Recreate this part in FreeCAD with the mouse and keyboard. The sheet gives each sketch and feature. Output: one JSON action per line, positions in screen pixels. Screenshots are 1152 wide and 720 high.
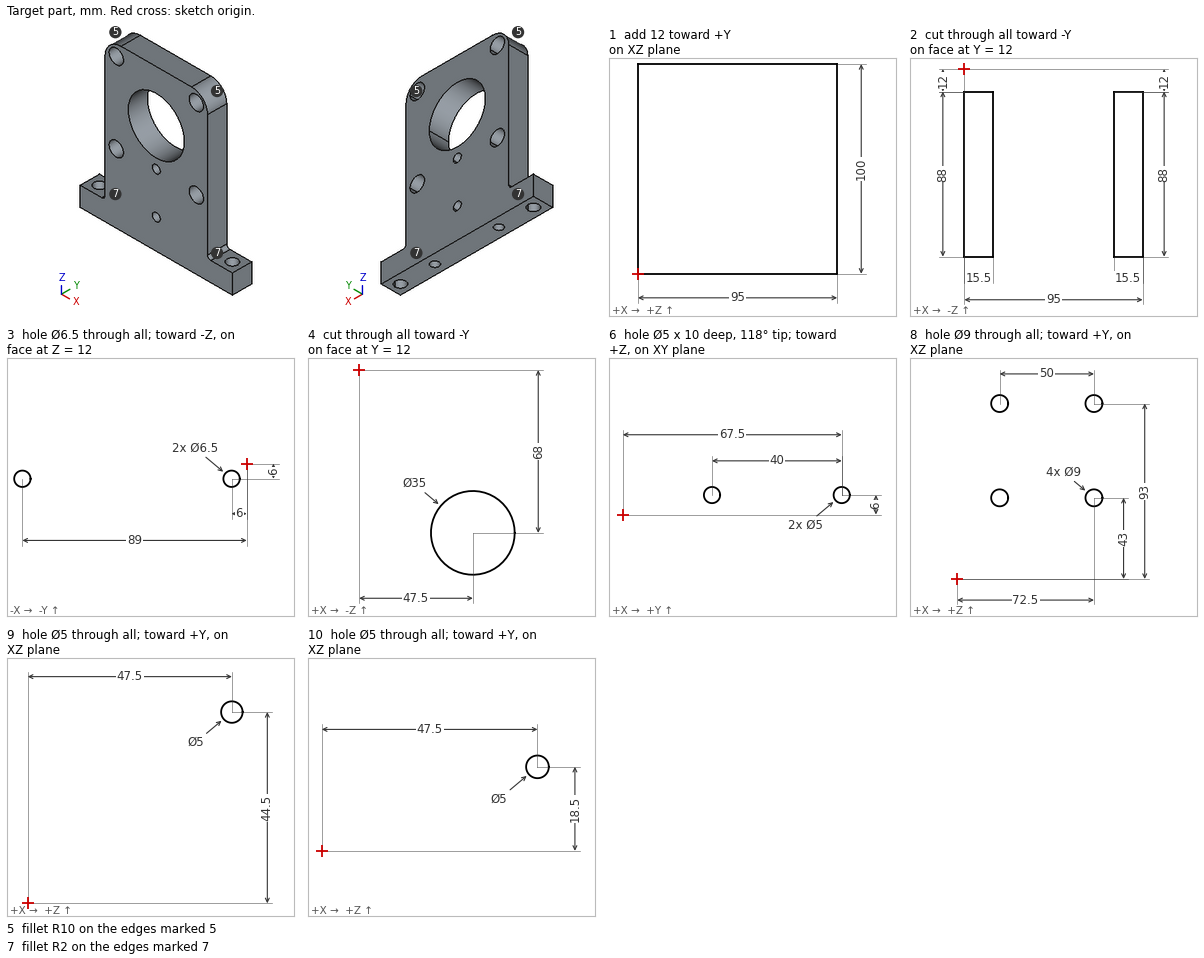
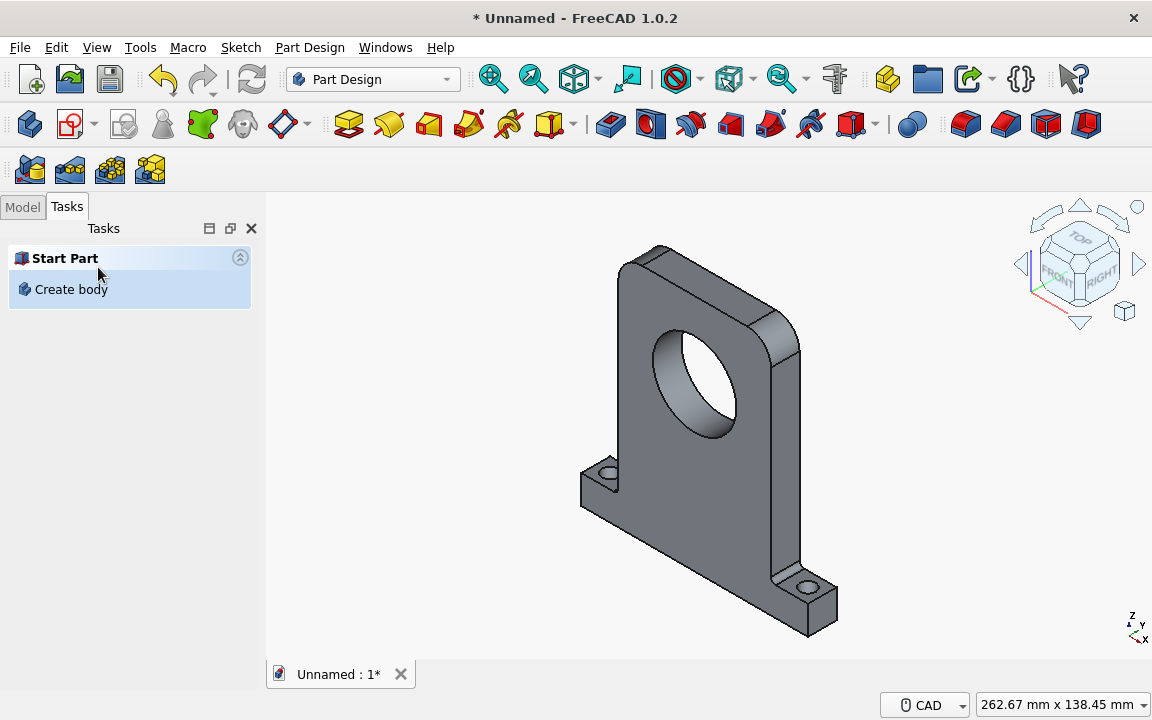
{"action": "left_click", "coordinate": [70, 124]}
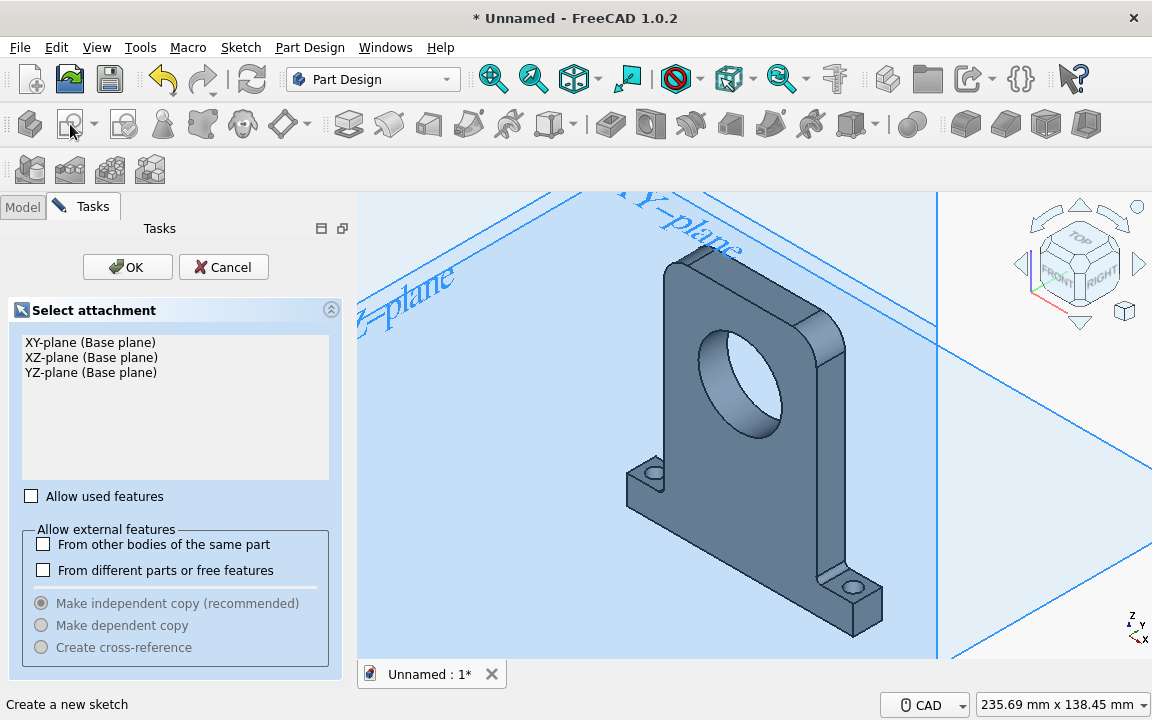
{"action": "left_click", "coordinate": [82, 358]}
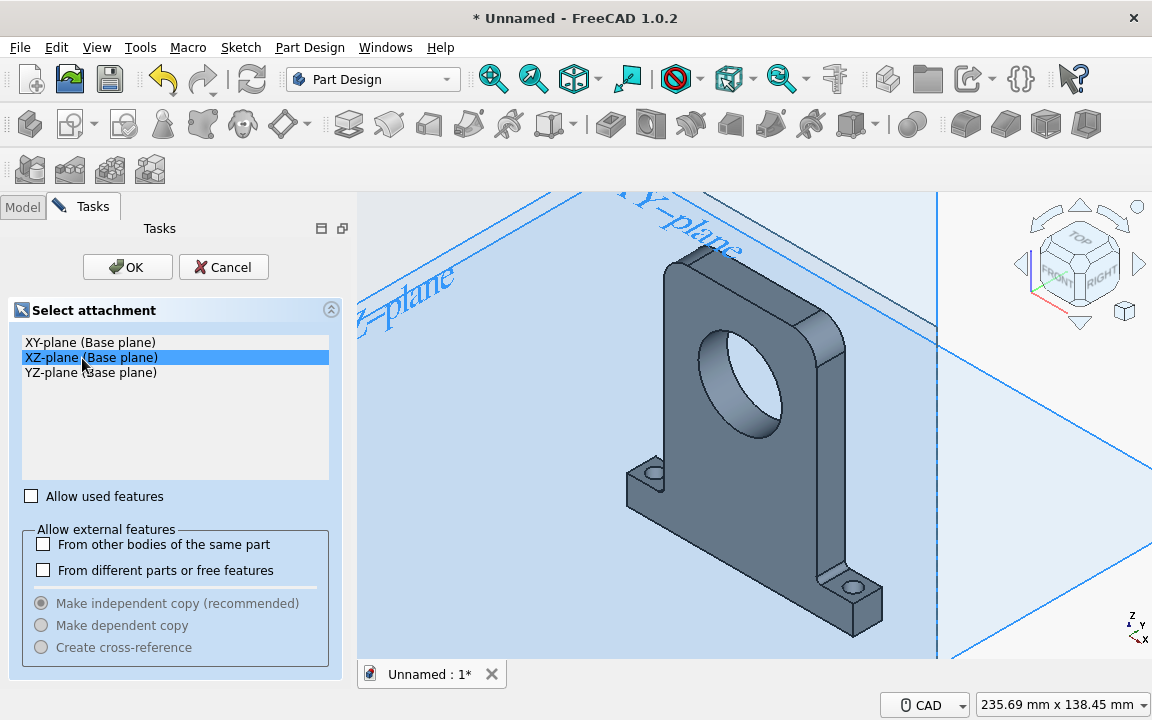
{"action": "left_click", "coordinate": [128, 267]}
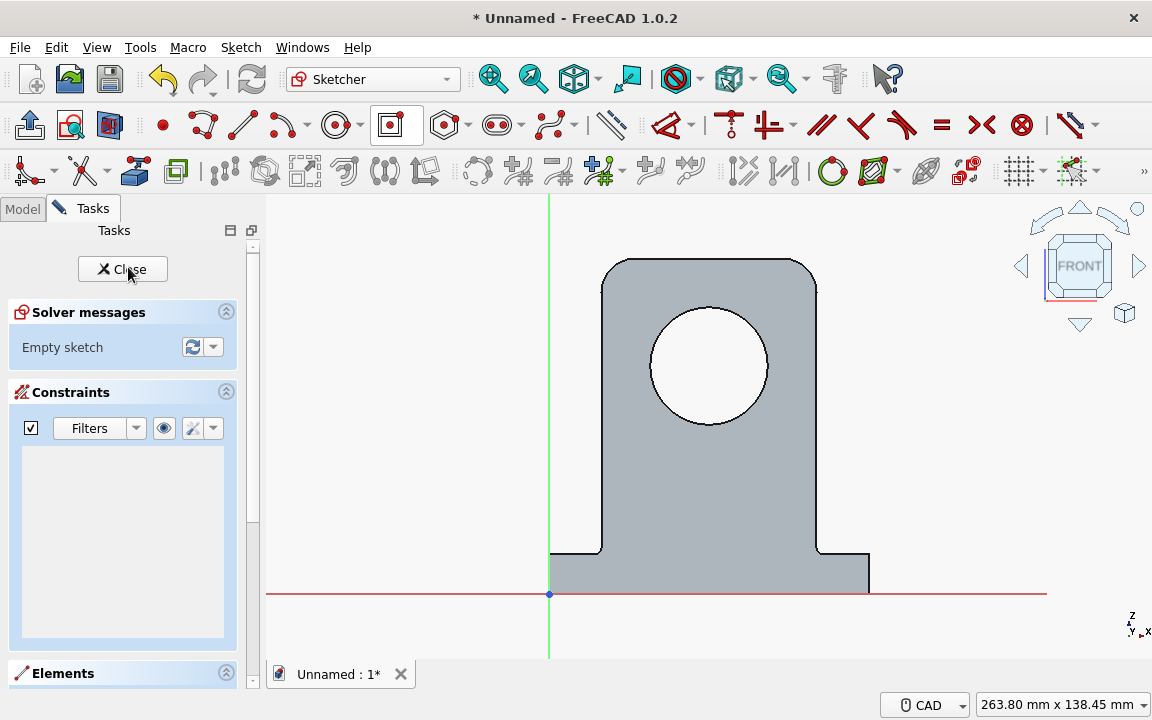
{"action": "left_click", "coordinate": [336, 126]}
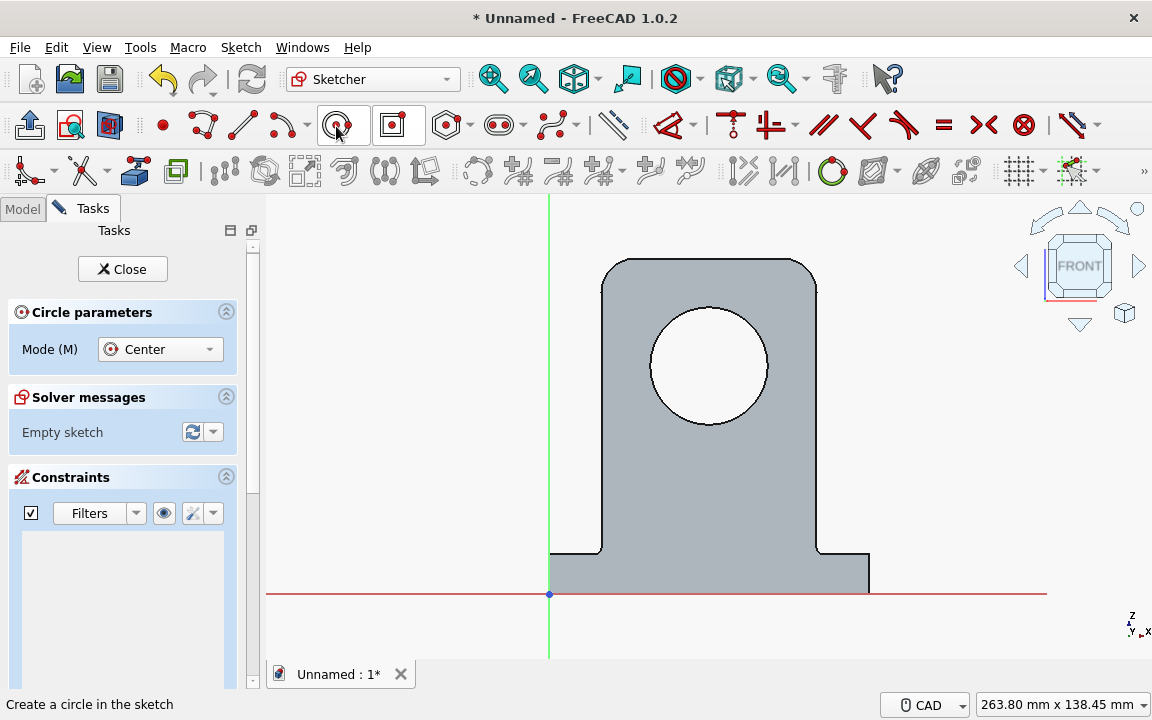
{"action": "scroll", "coordinate": [793, 450], "scroll_direction": "up", "scroll_amount": 3}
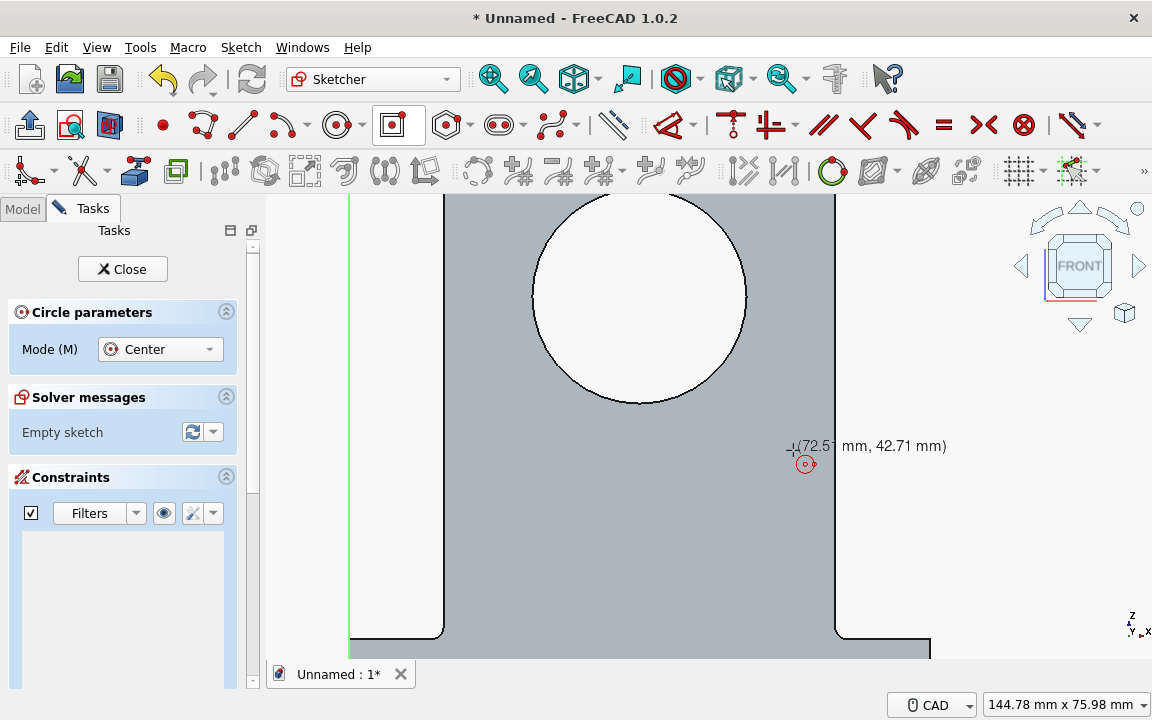
{"action": "left_click", "coordinate": [792, 450]}
{"action": "left_click", "coordinate": [812, 430]}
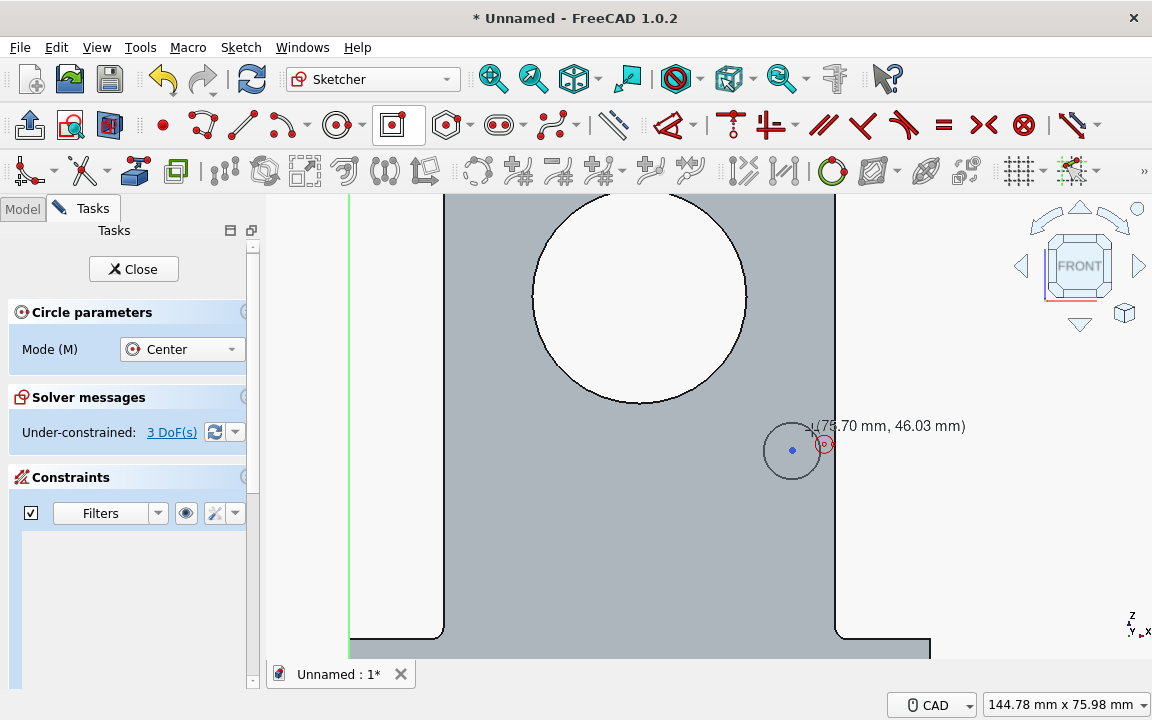
{"action": "scroll", "coordinate": [686, 436], "scroll_direction": "down", "scroll_amount": 4}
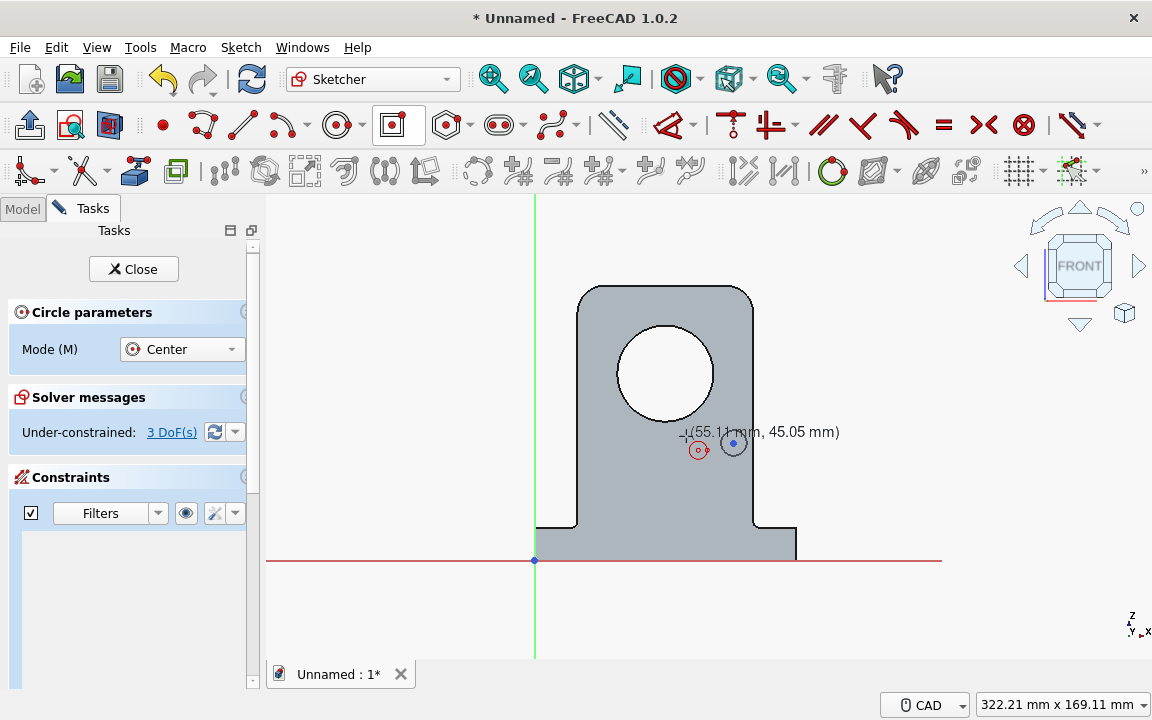
{"action": "scroll", "coordinate": [734, 305], "scroll_direction": "up", "scroll_amount": 4}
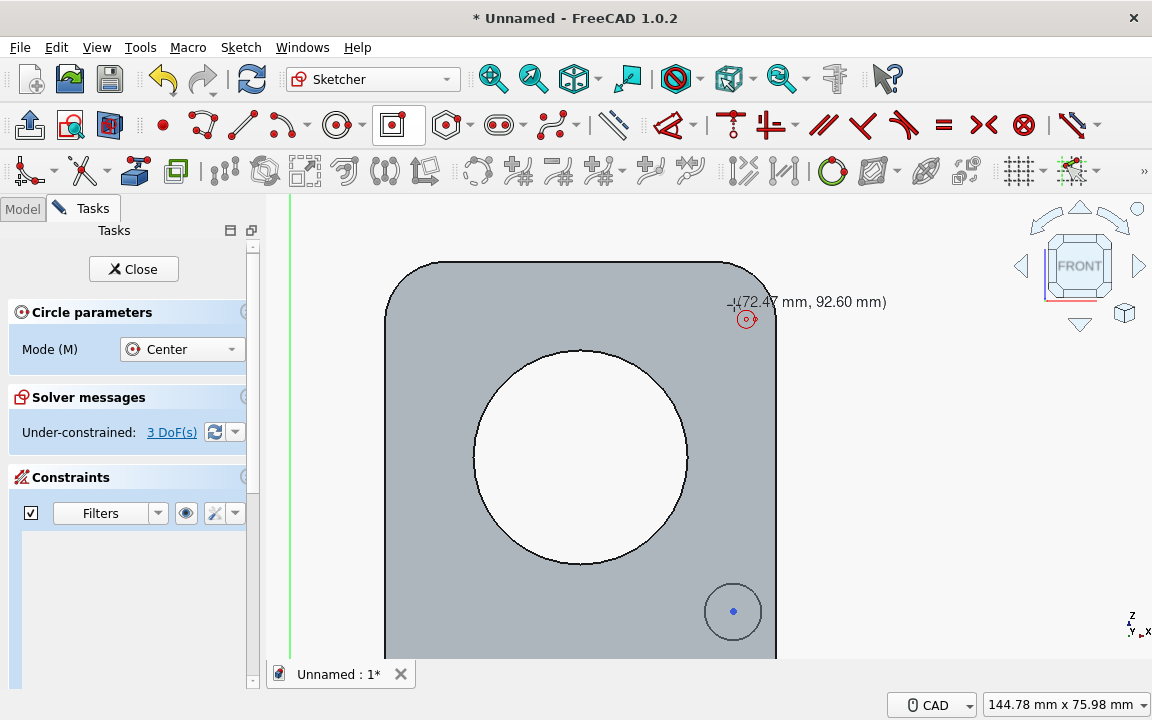
{"action": "left_click", "coordinate": [734, 304]}
{"action": "left_click", "coordinate": [753, 285]}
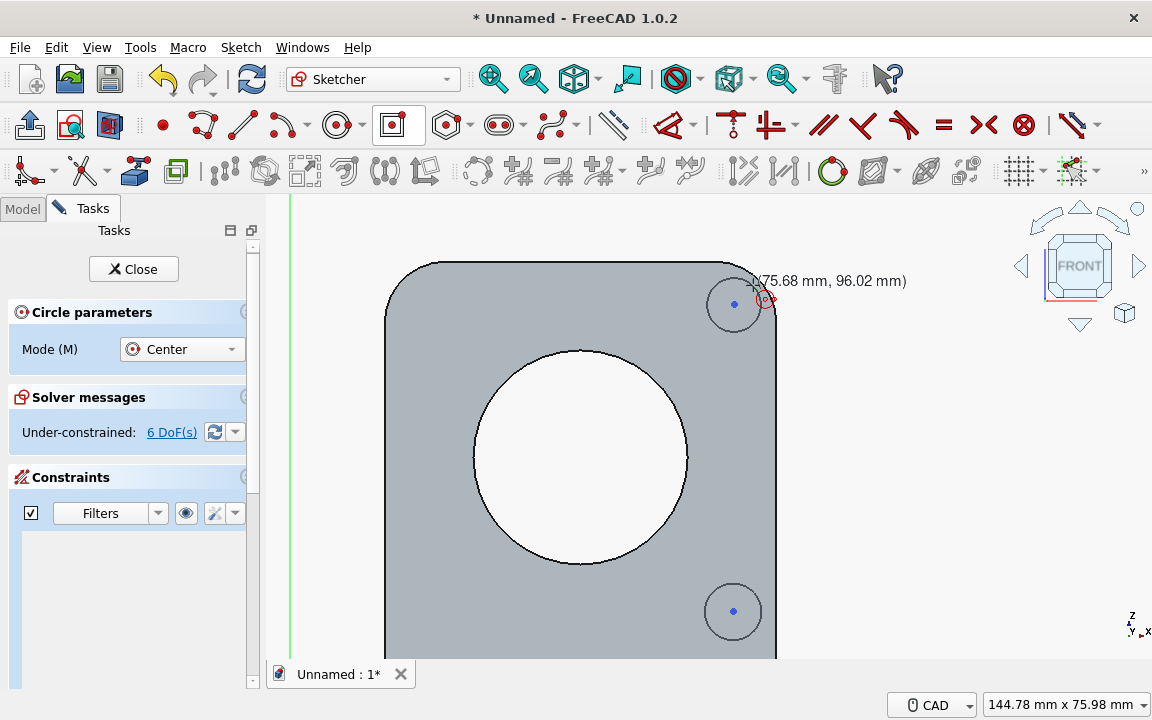
{"action": "left_click", "coordinate": [428, 304]}
{"action": "left_click", "coordinate": [447, 285]}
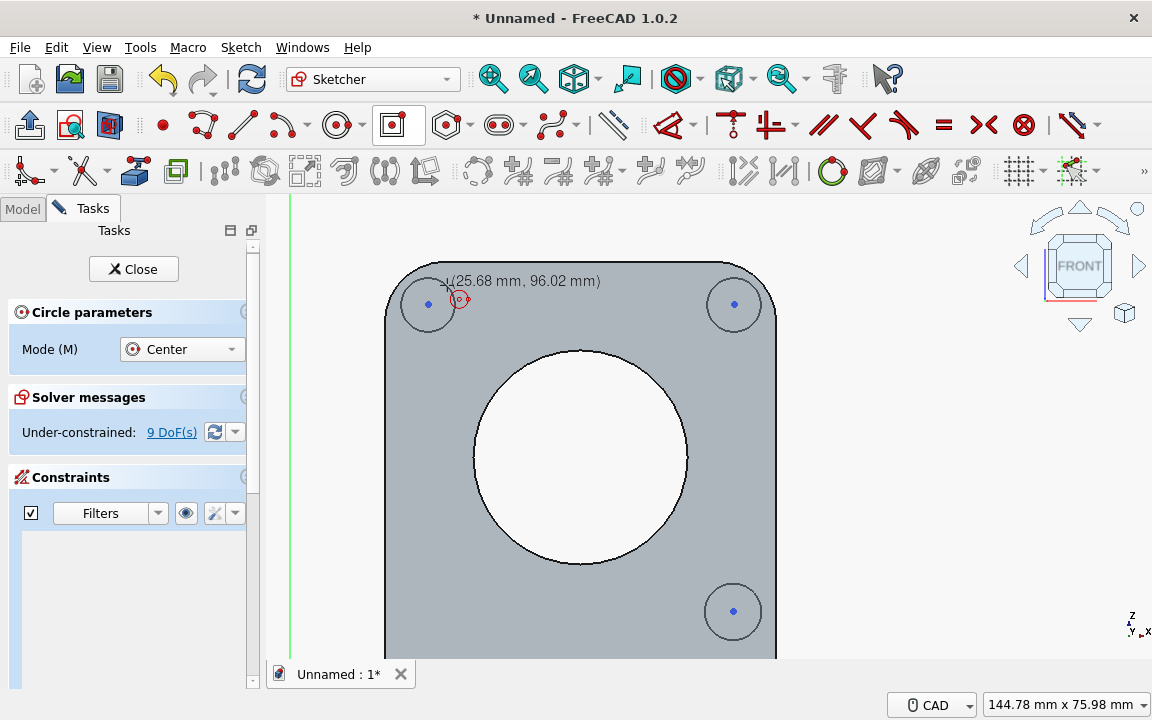
{"action": "left_click", "coordinate": [428, 610]}
{"action": "left_click", "coordinate": [447, 591]}
{"action": "key", "text": "Escape"}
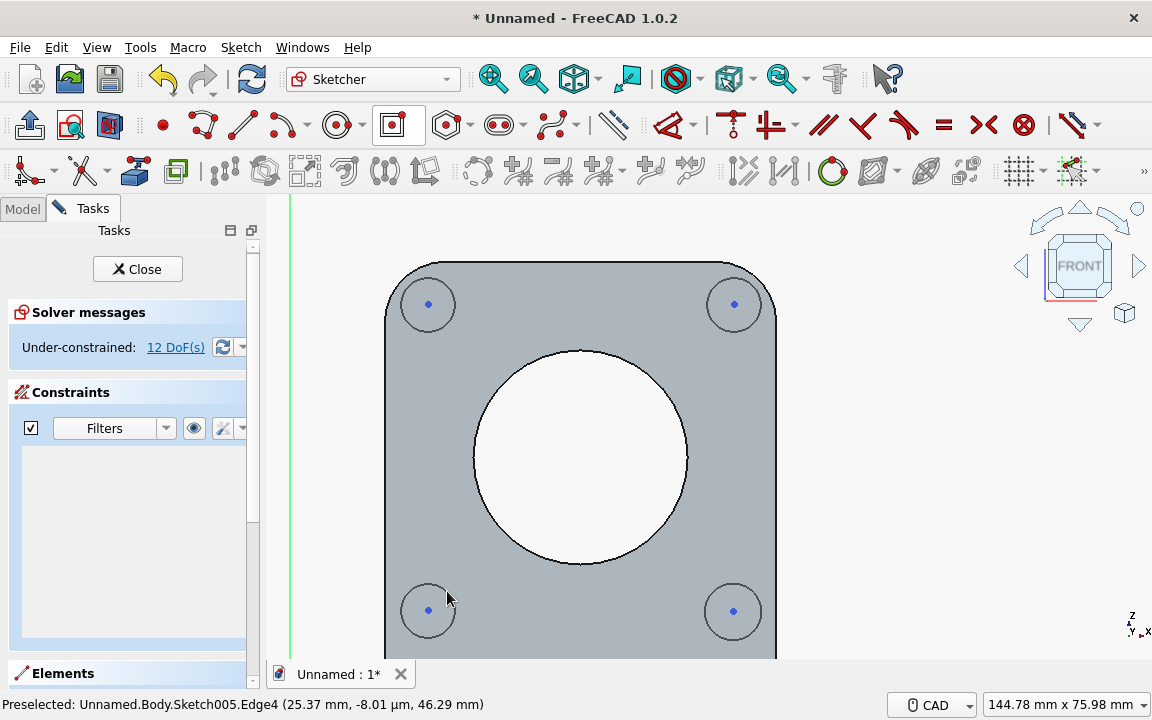
{"action": "left_click", "coordinate": [753, 592]}